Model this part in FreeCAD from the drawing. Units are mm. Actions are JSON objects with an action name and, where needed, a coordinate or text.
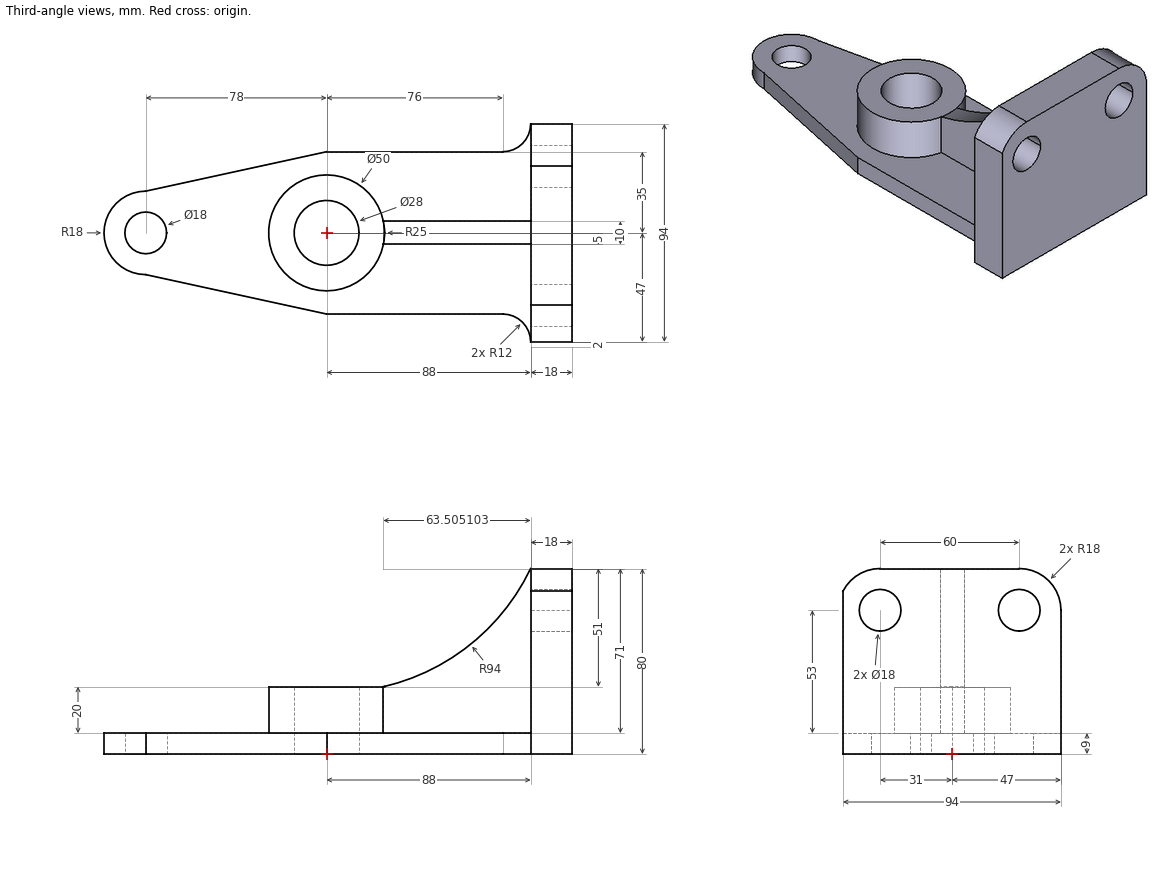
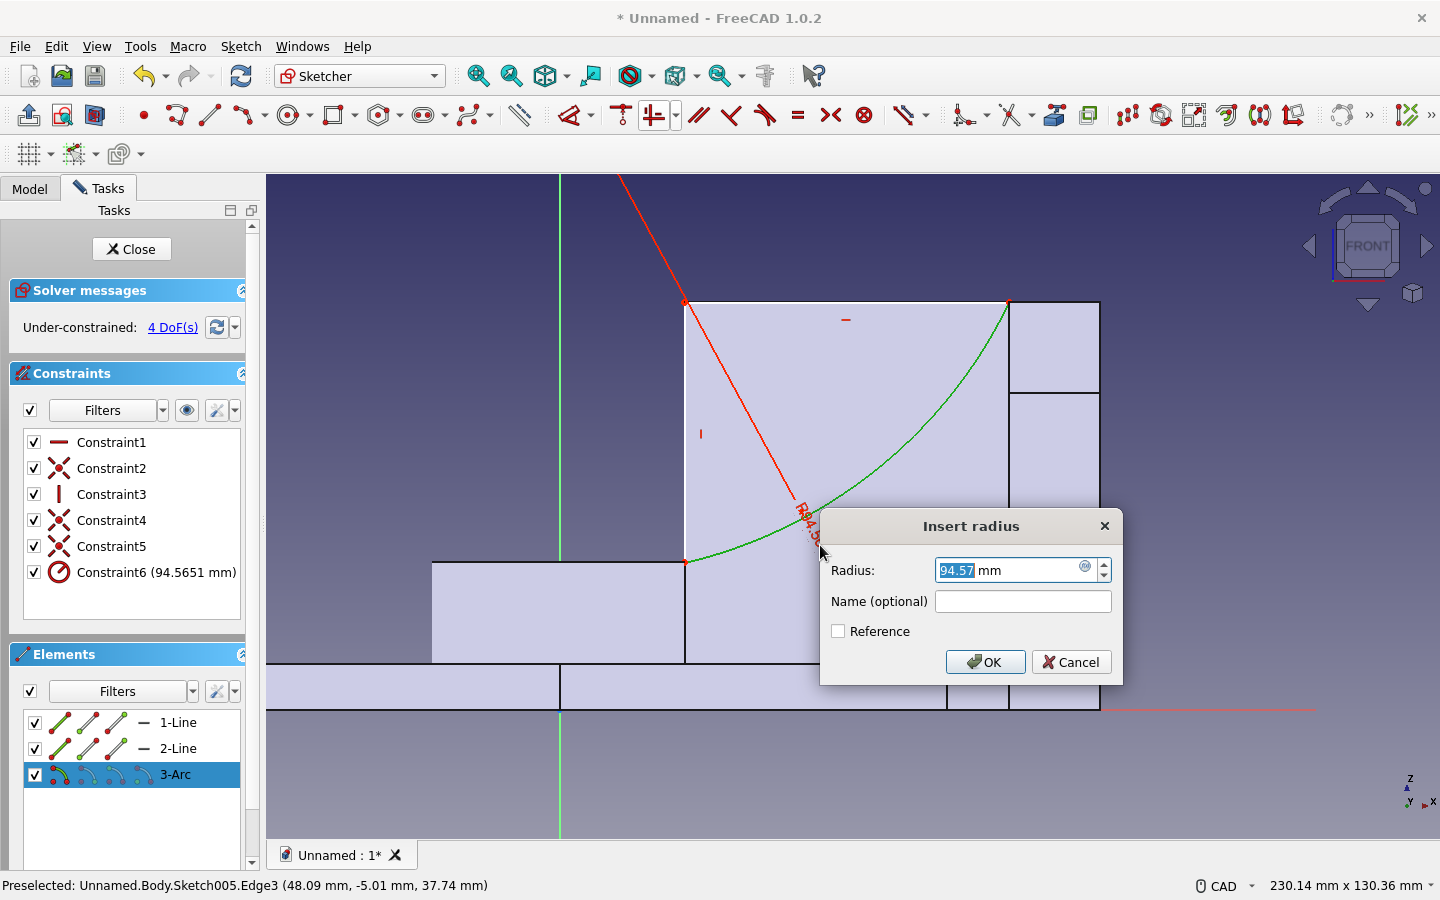
{"action": "type", "text": "94"}
{"action": "key", "text": "Return"}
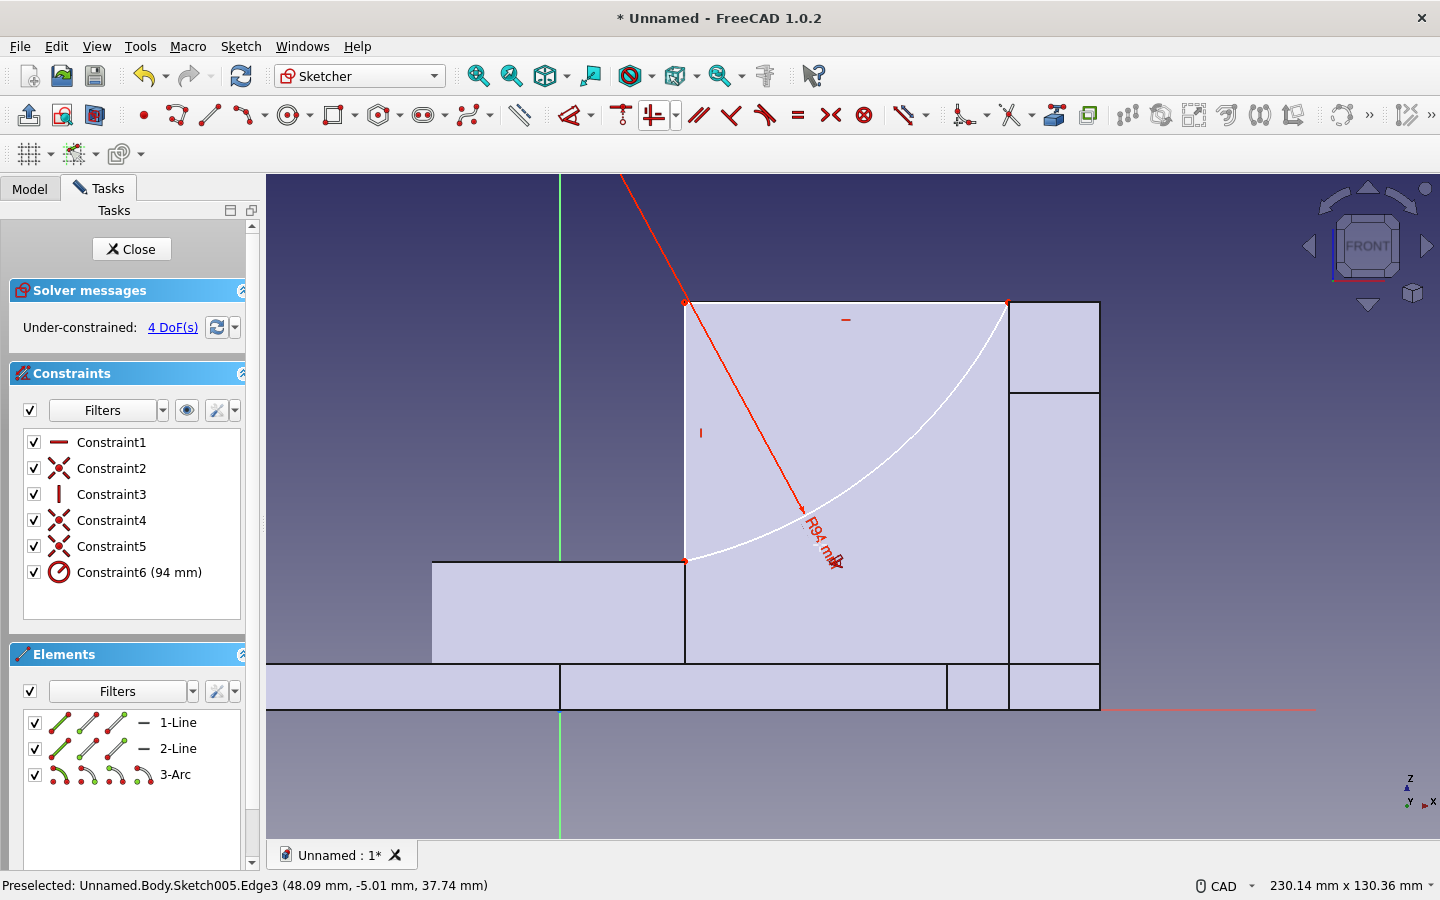
{"action": "left_click", "coordinate": [685, 380]}
{"action": "left_click", "coordinate": [651, 432]}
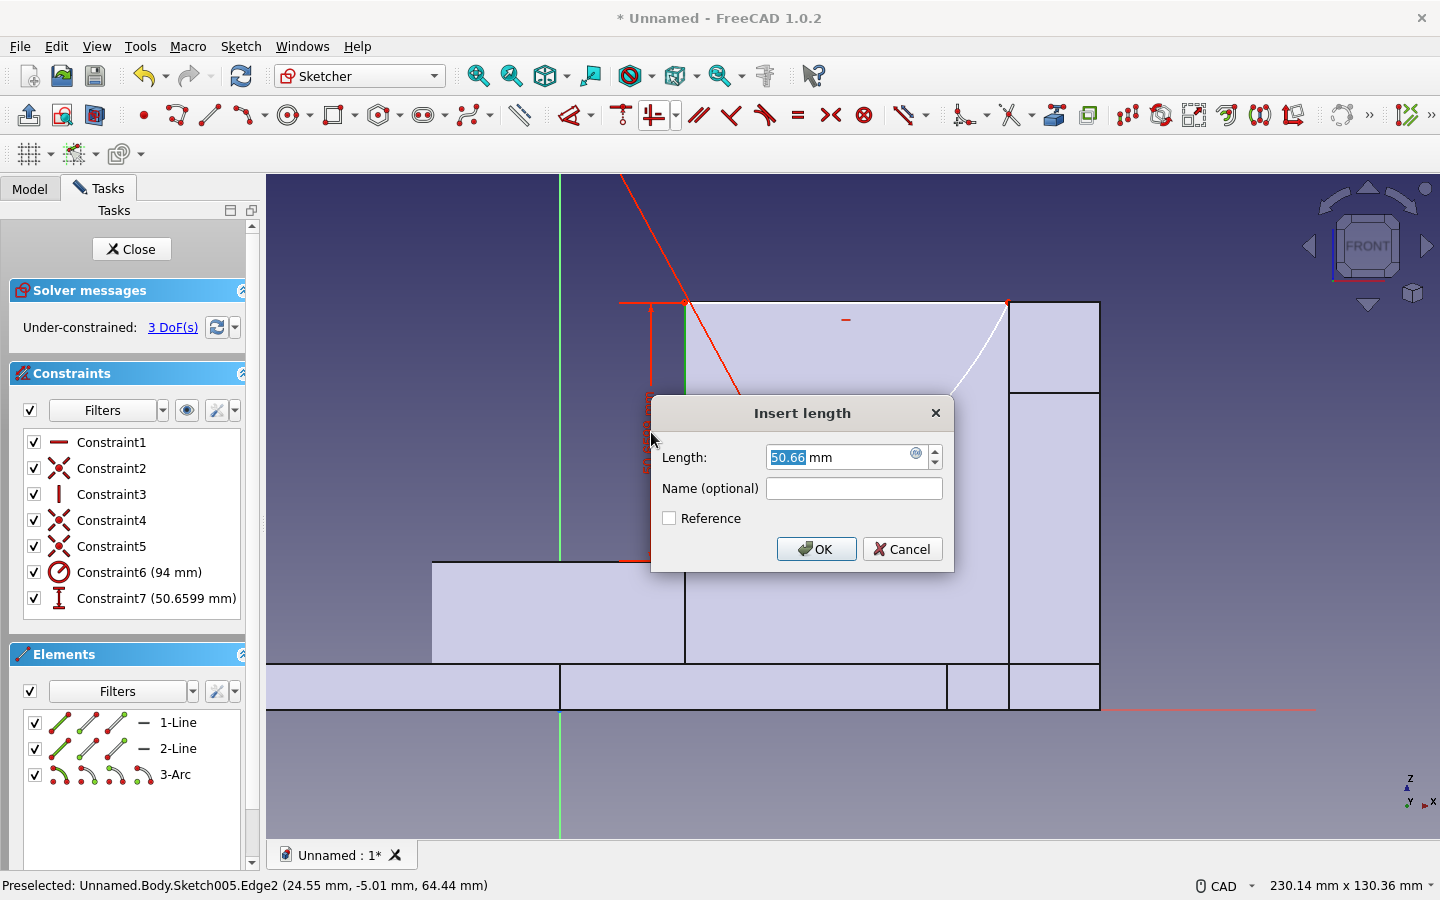
{"action": "type", "text": "51"}
{"action": "key", "text": "Return"}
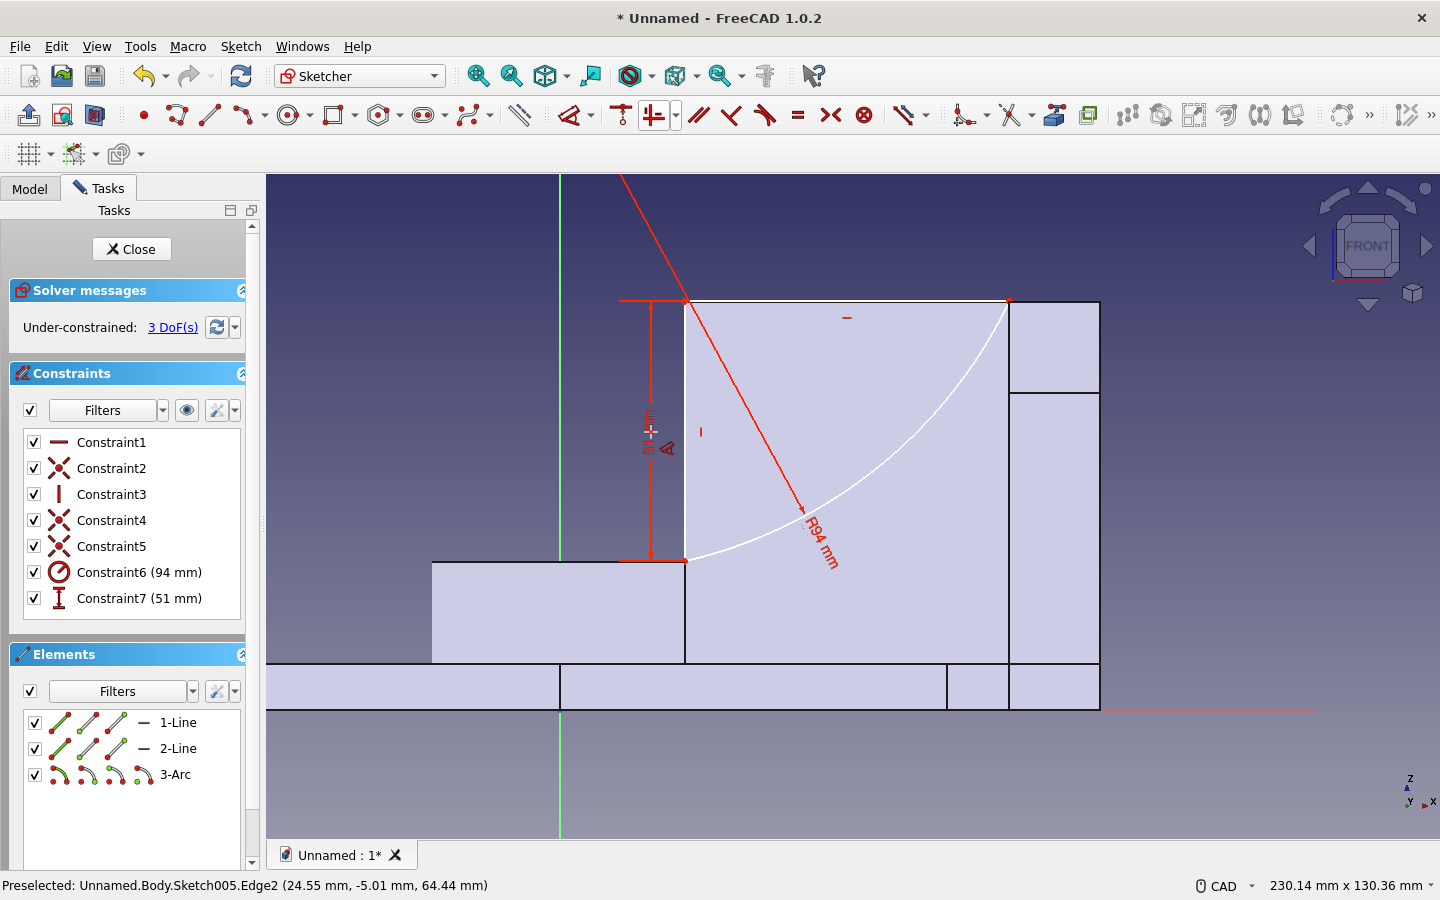
{"action": "left_click", "coordinate": [1009, 301]}
{"action": "left_click", "coordinate": [785, 267]}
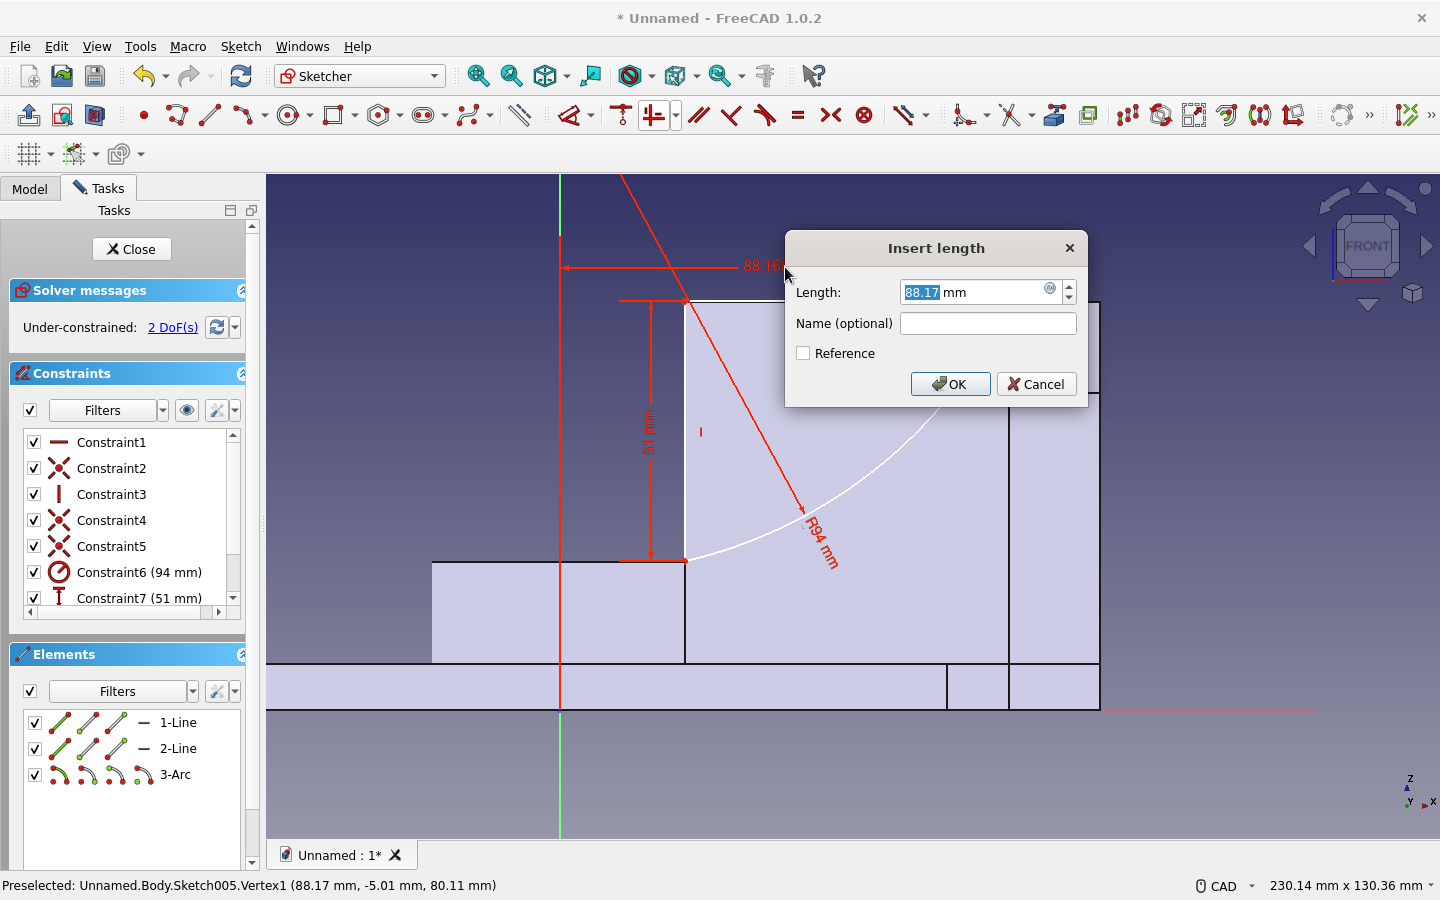
{"action": "type", "text": "88"}
{"action": "key", "text": "Return"}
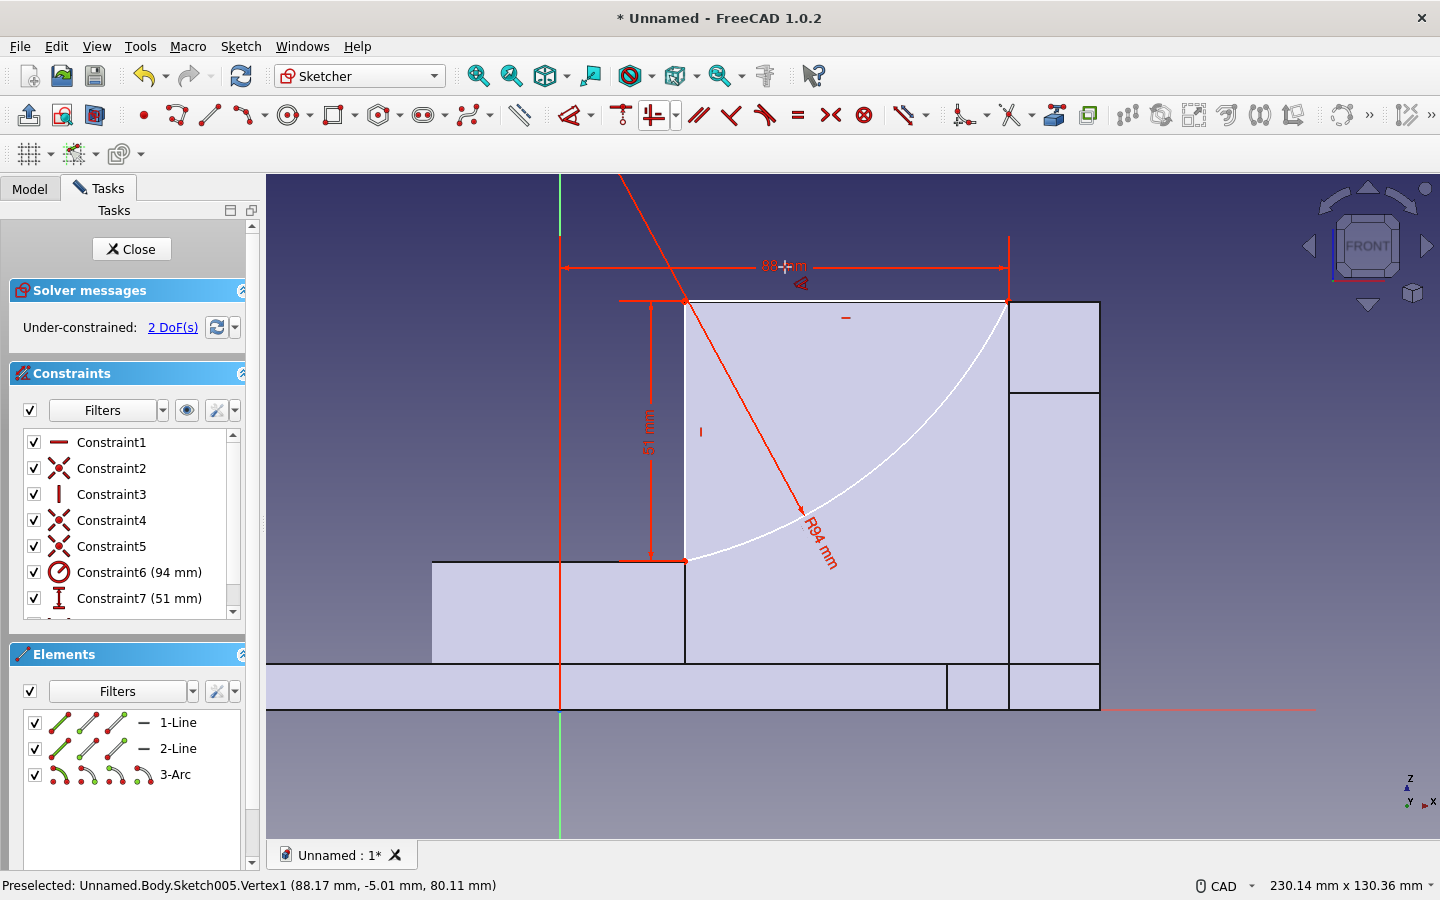
{"action": "left_click", "coordinate": [1009, 301]}
{"action": "left_click", "coordinate": [1043, 505]}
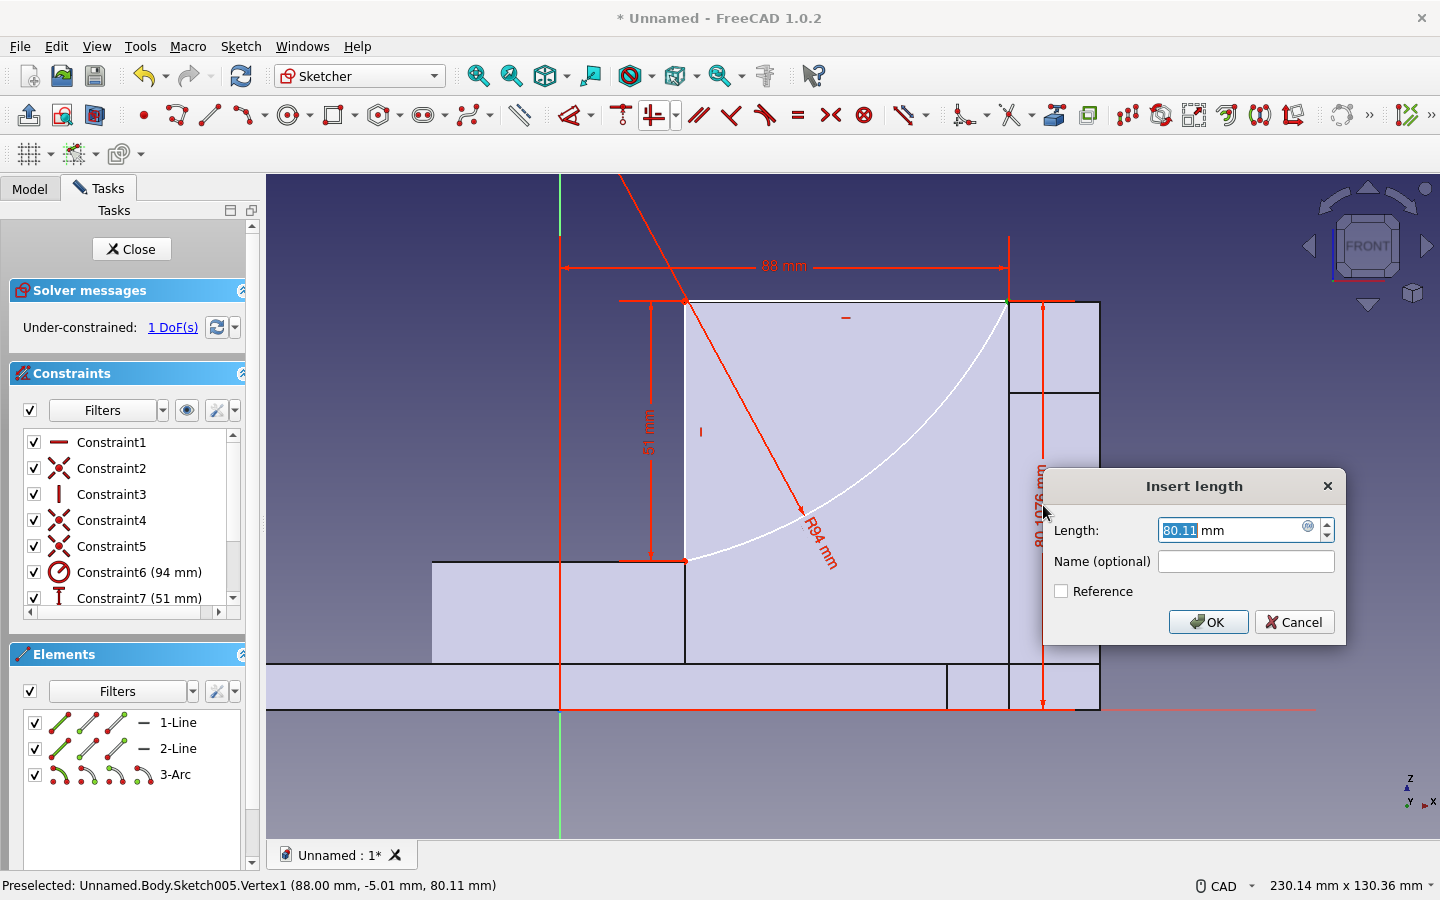
{"action": "type", "text": "80"}
{"action": "key", "text": "Return"}